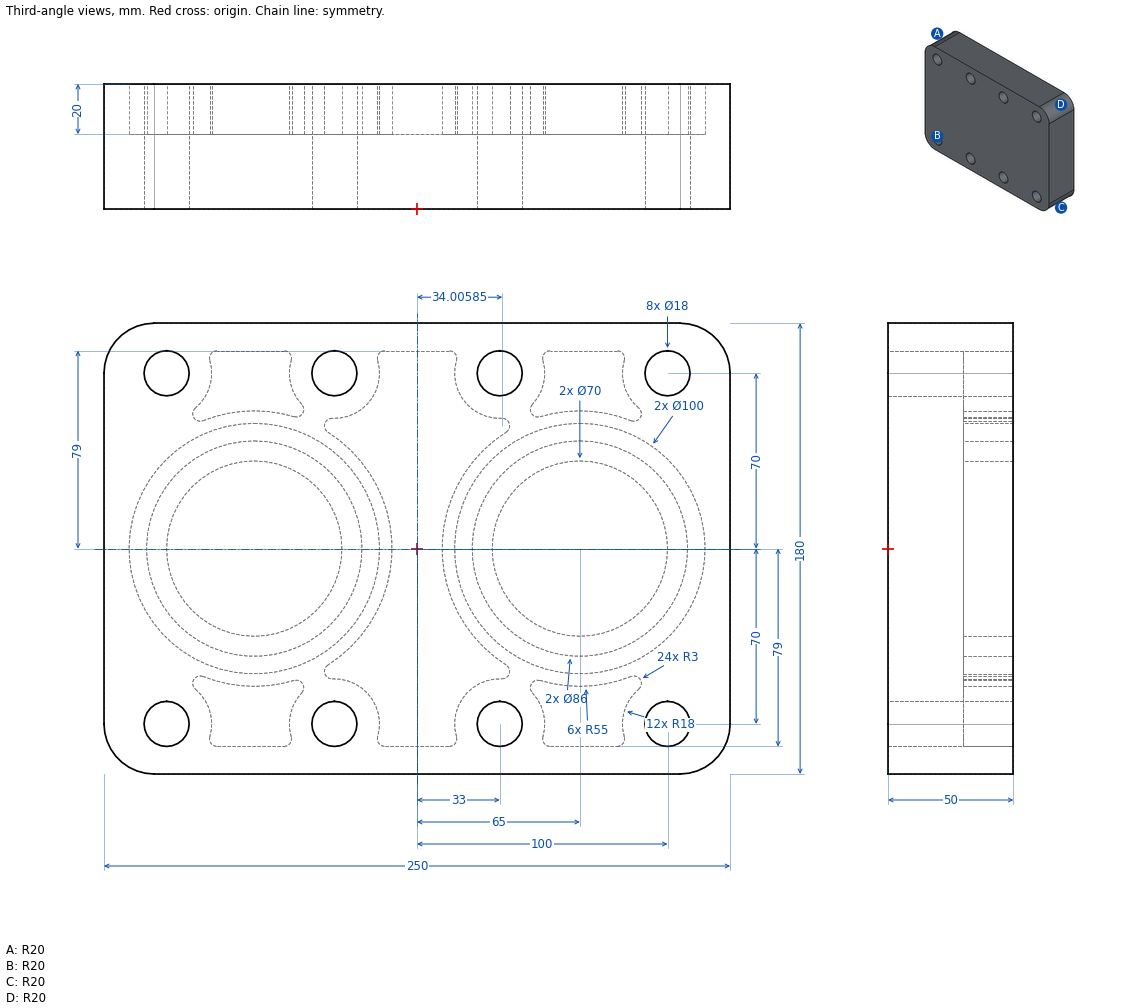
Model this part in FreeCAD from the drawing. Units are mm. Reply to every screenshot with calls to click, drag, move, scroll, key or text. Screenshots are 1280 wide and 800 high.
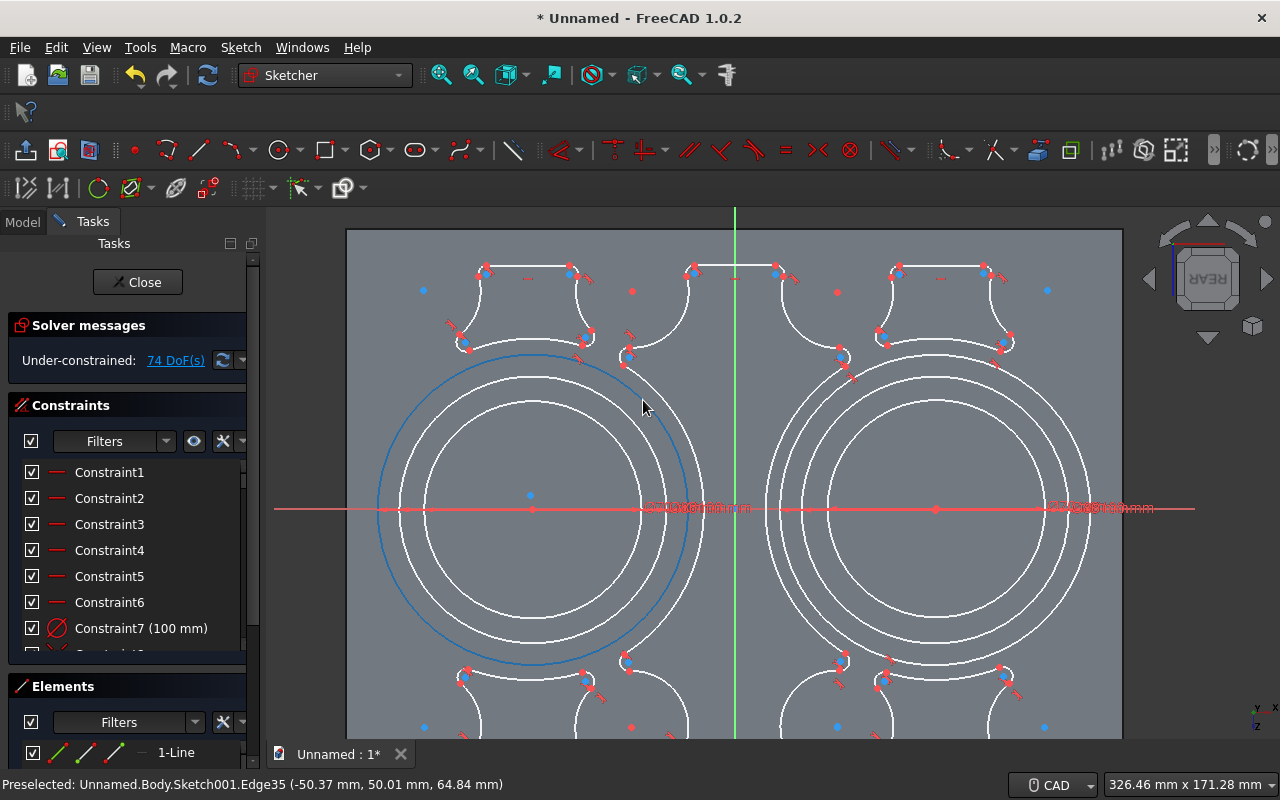
click(642, 400)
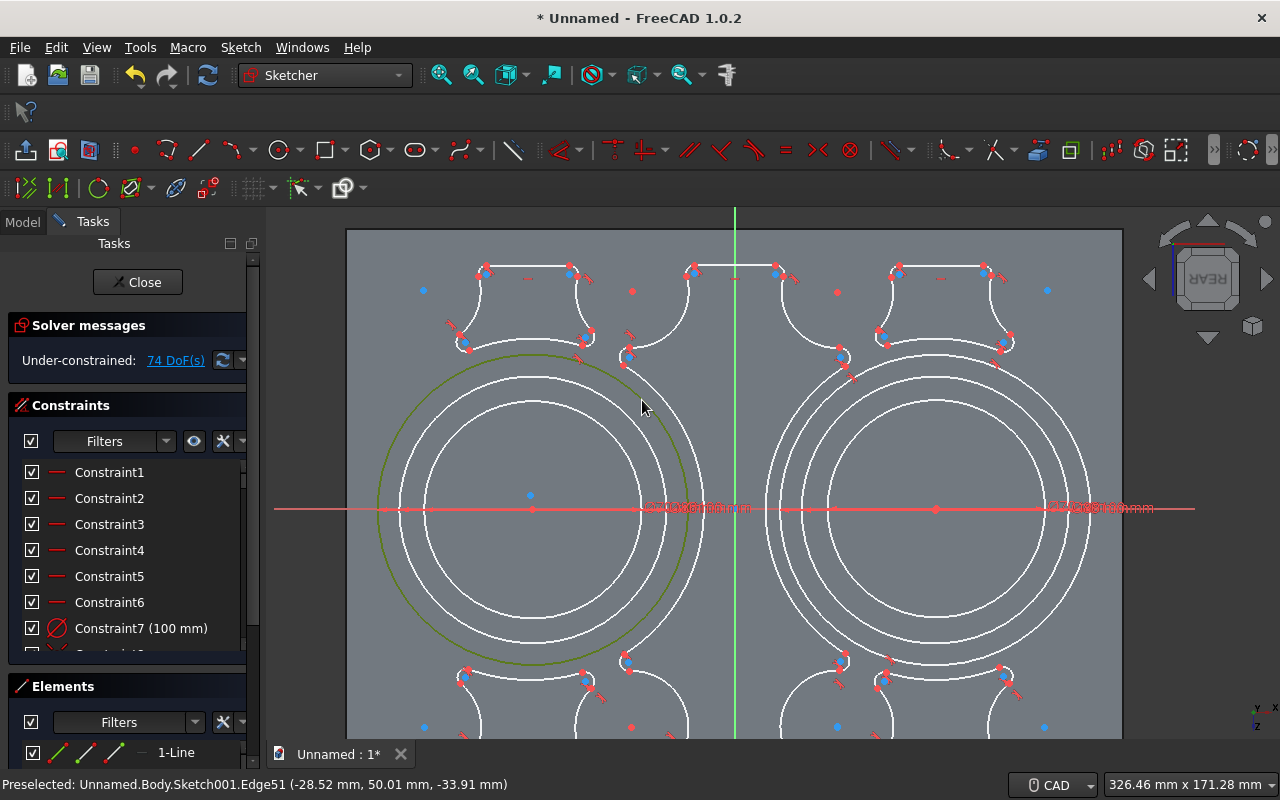
click(502, 678)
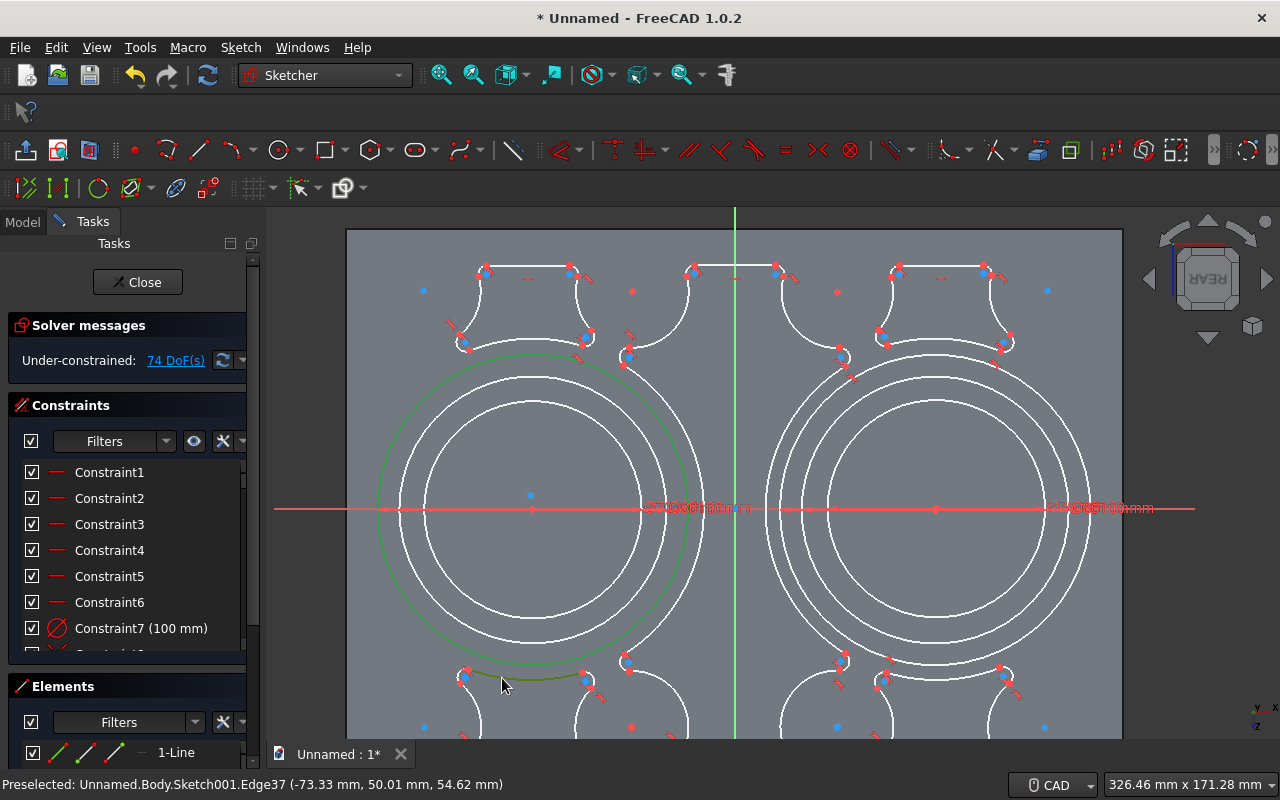
click(614, 150)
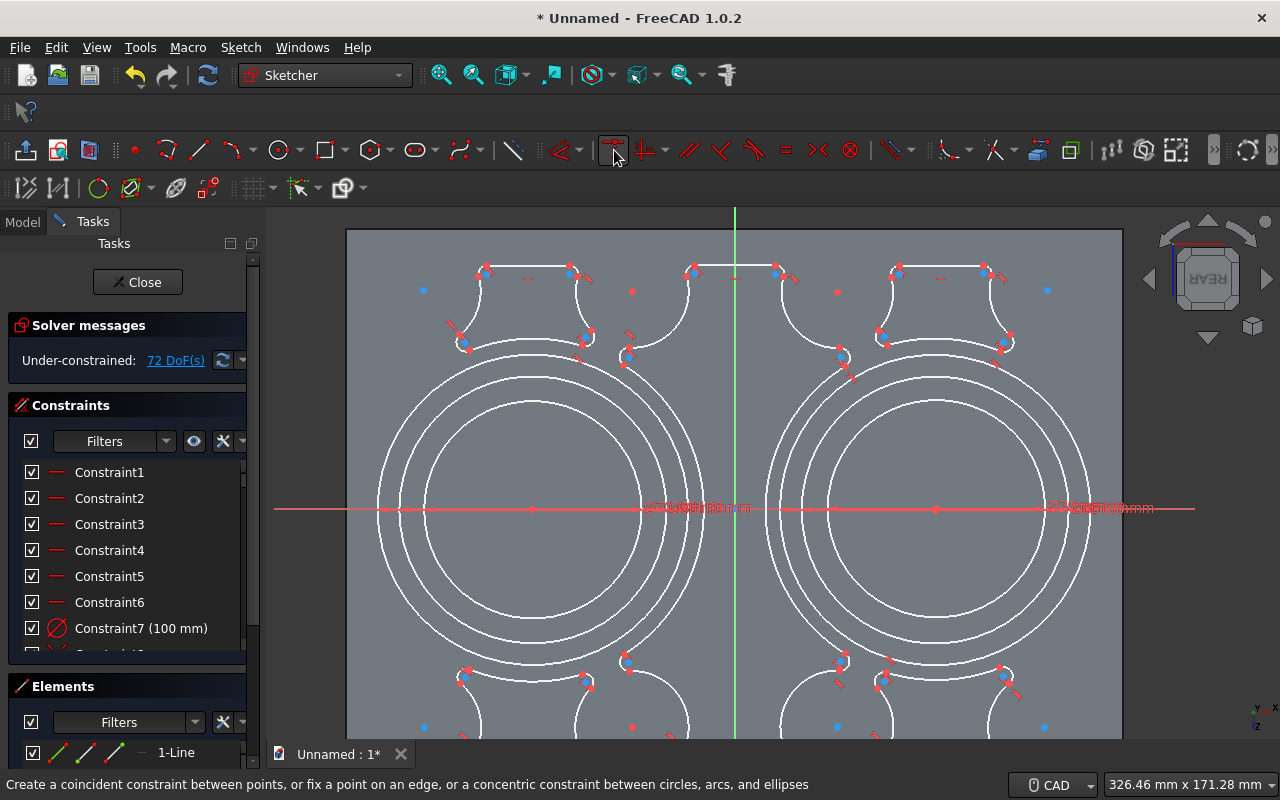
click(1045, 400)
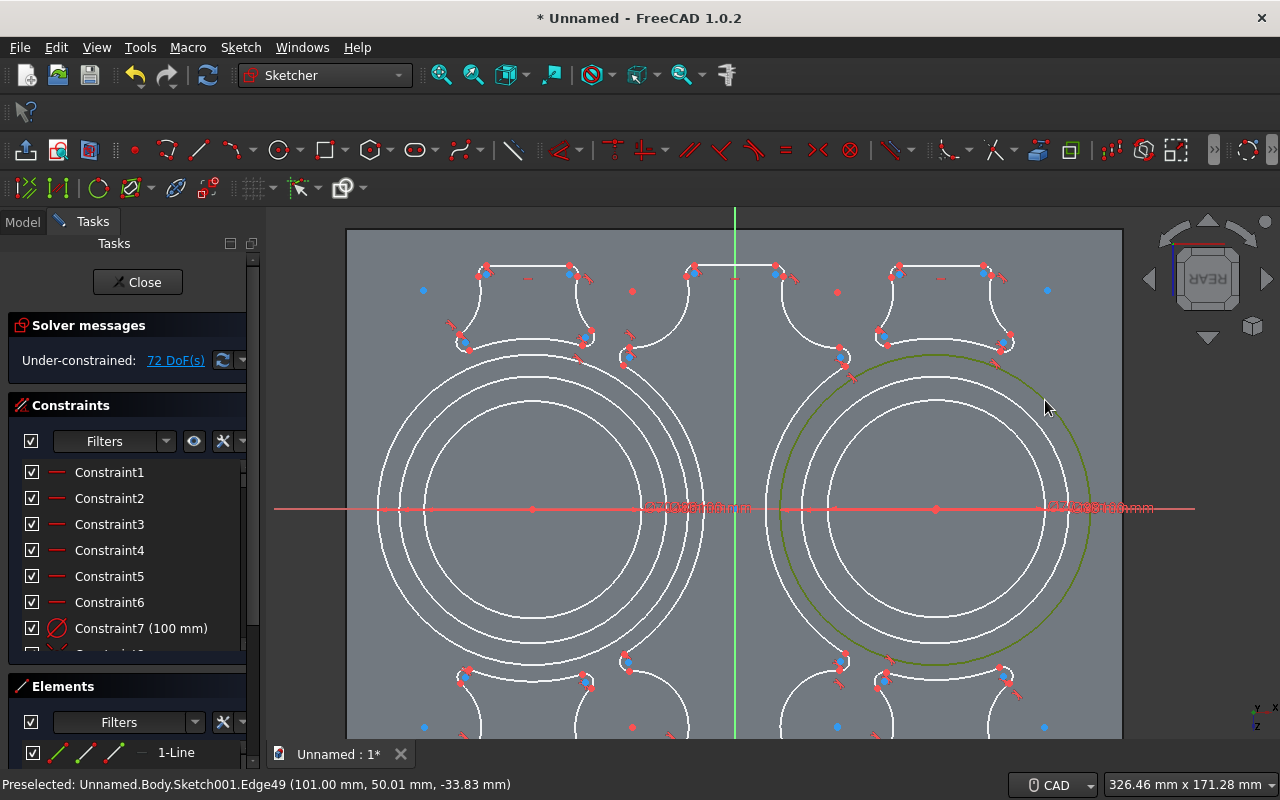
click(921, 679)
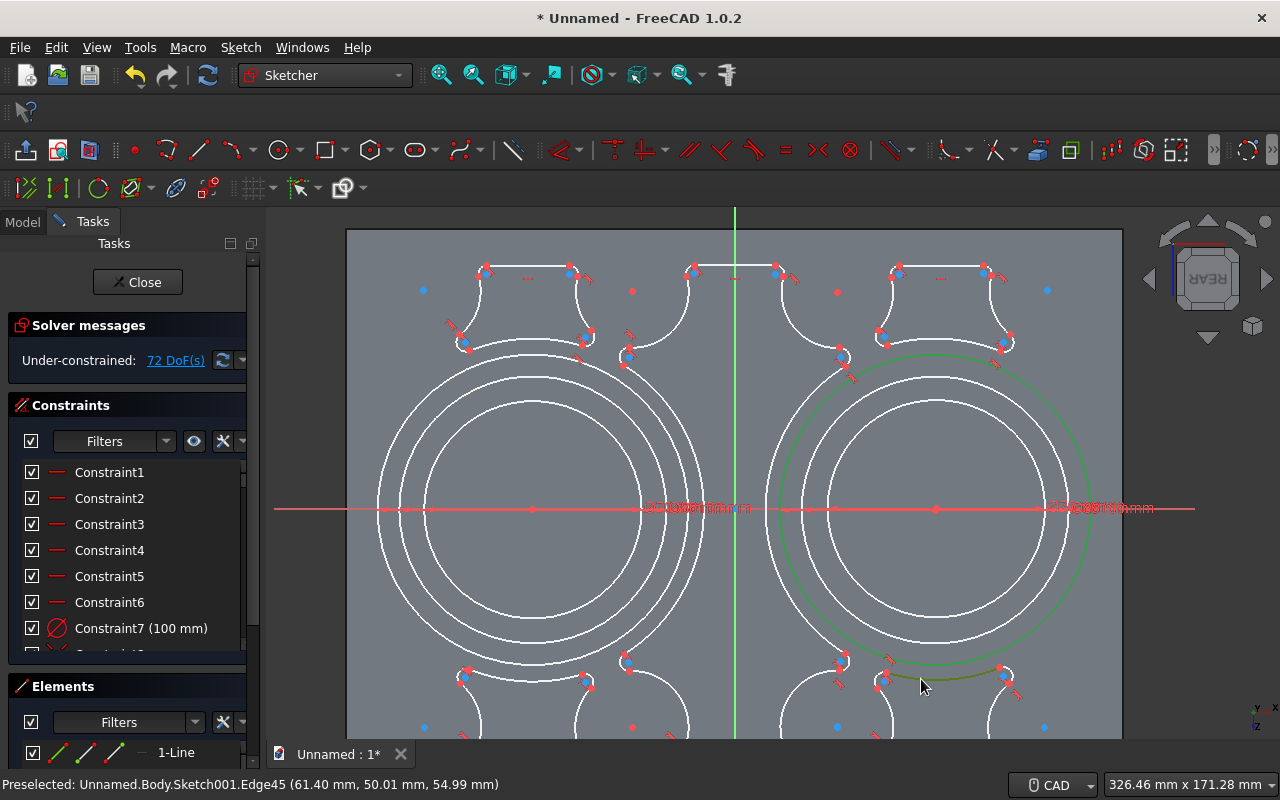
click(614, 150)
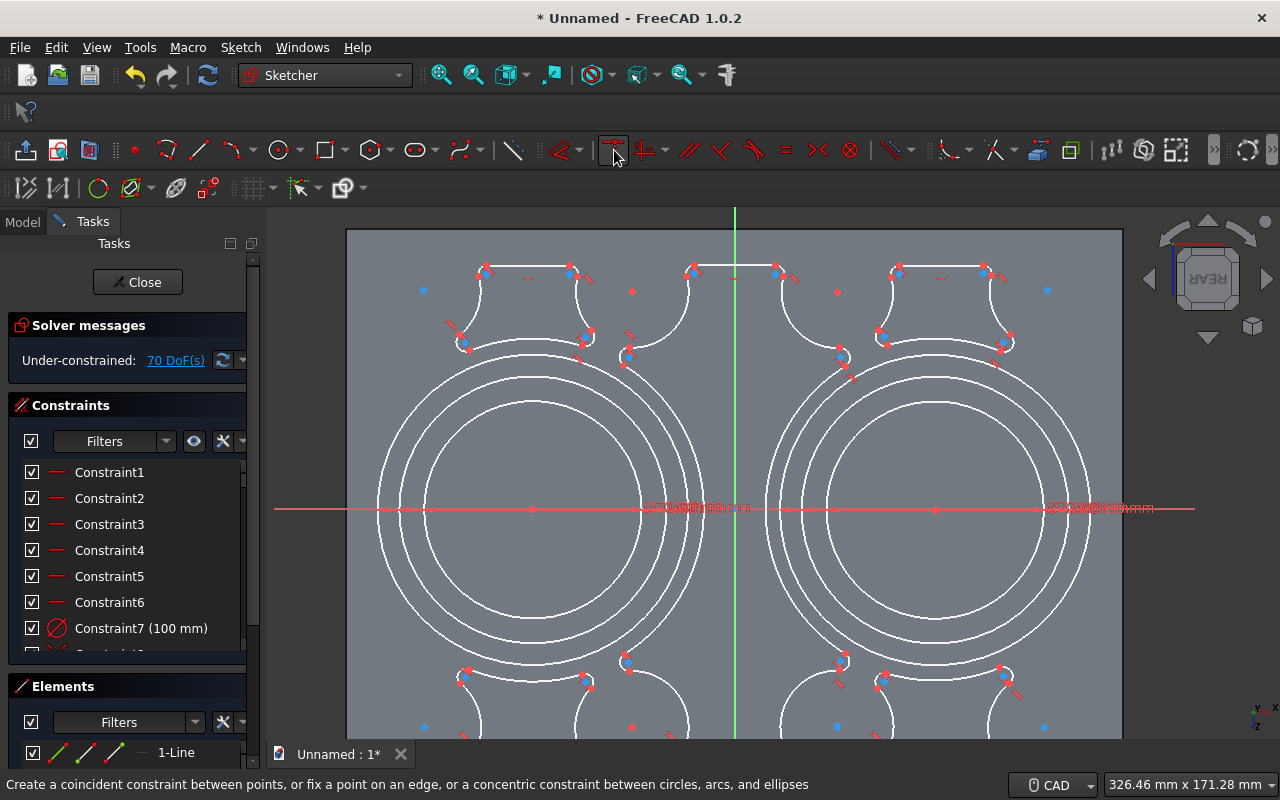
click(809, 678)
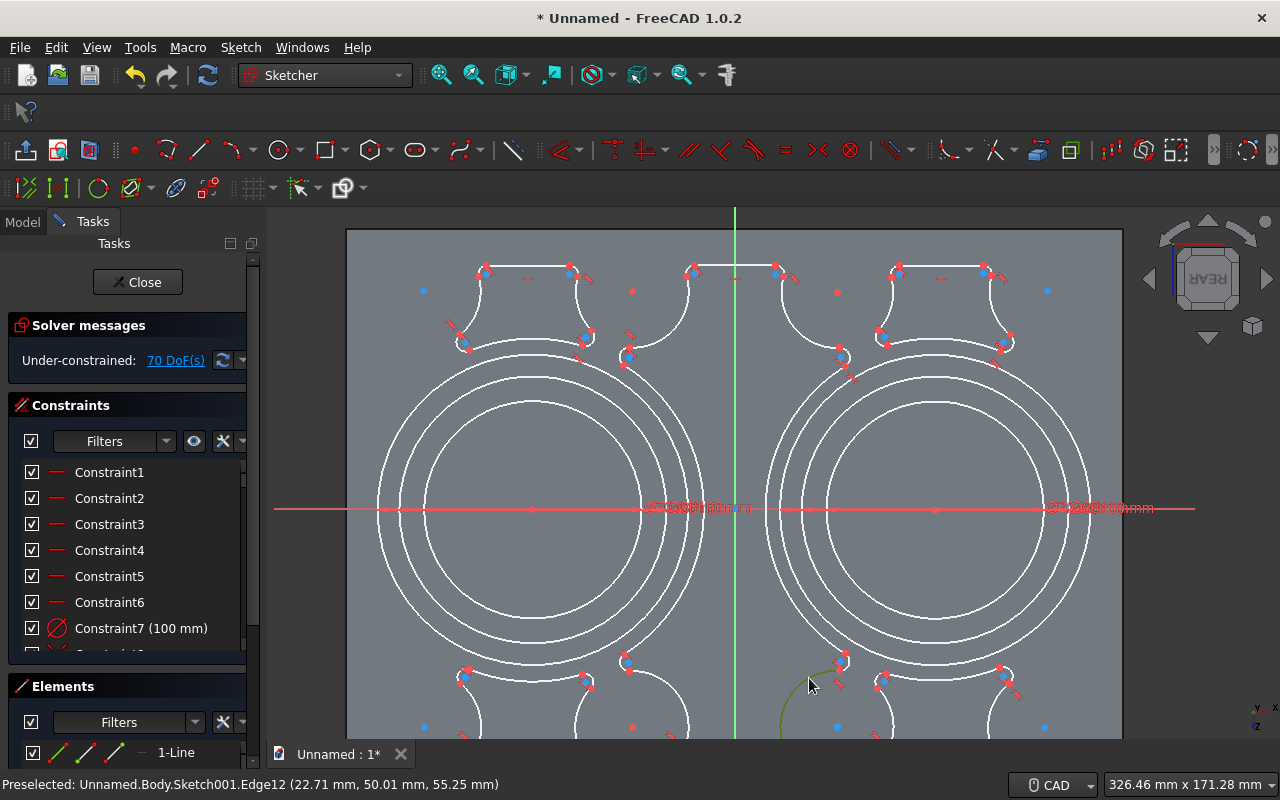
click(888, 702)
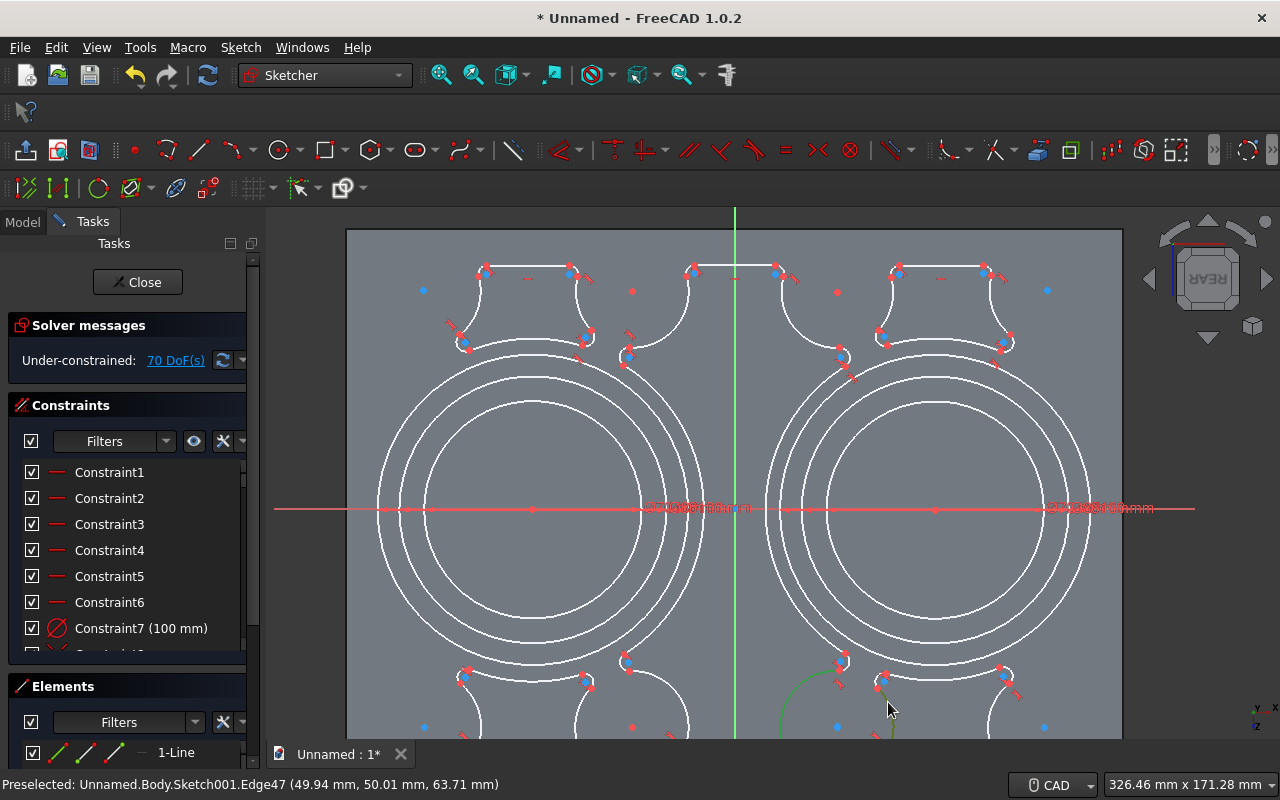
click(614, 150)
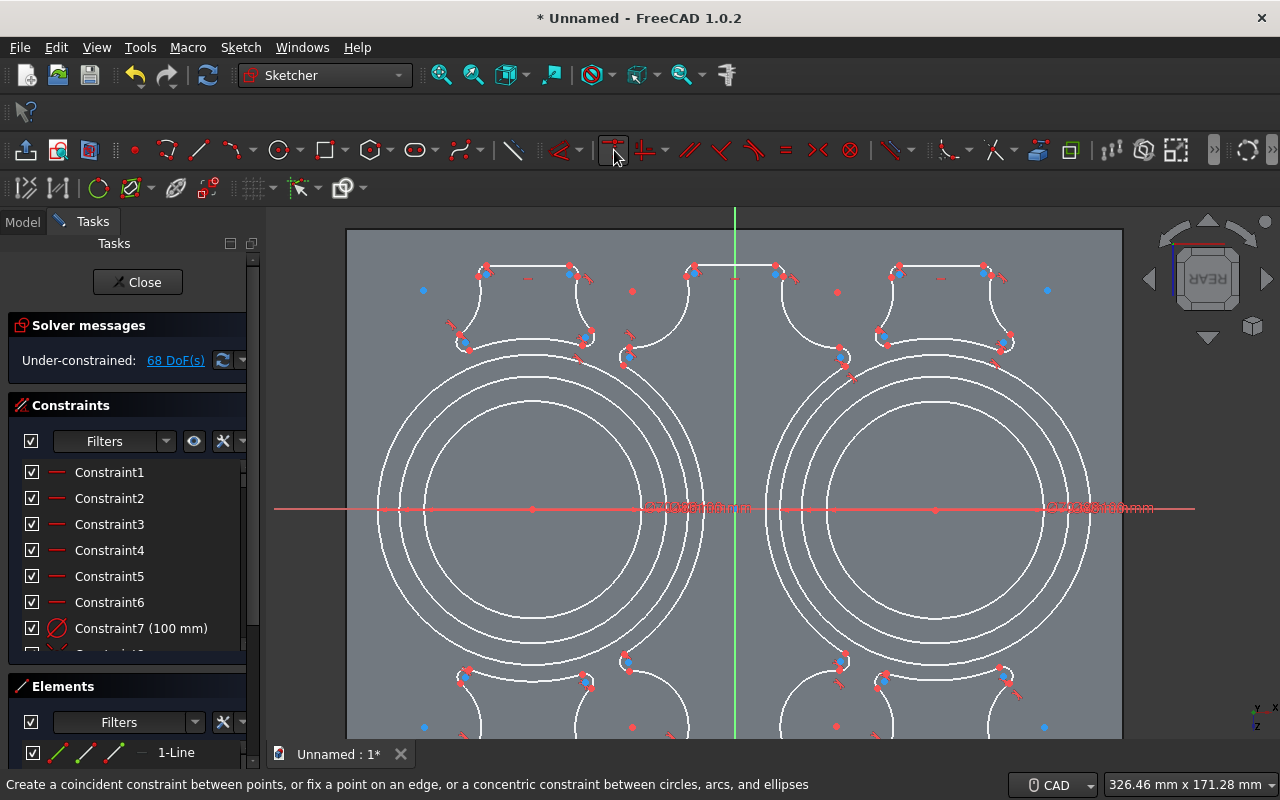
scroll(893, 269, up, 3)